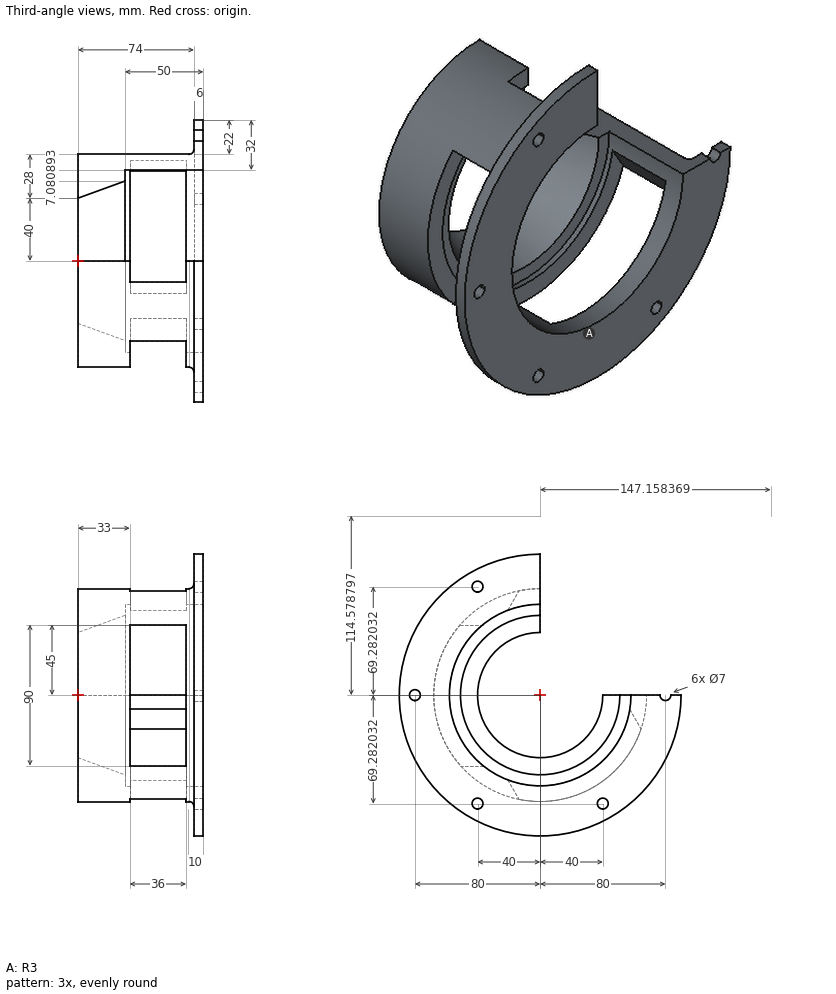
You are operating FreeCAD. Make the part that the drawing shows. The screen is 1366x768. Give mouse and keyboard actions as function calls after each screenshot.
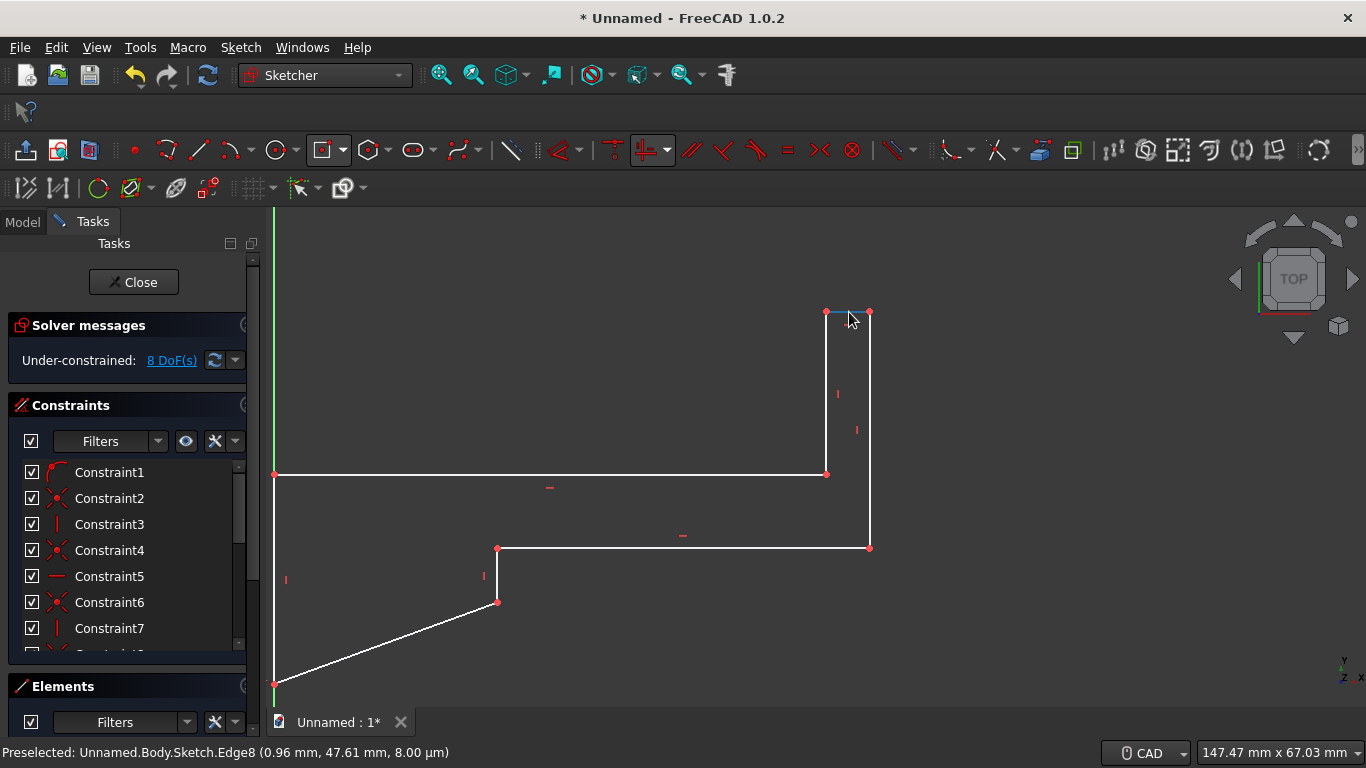
click(848, 312)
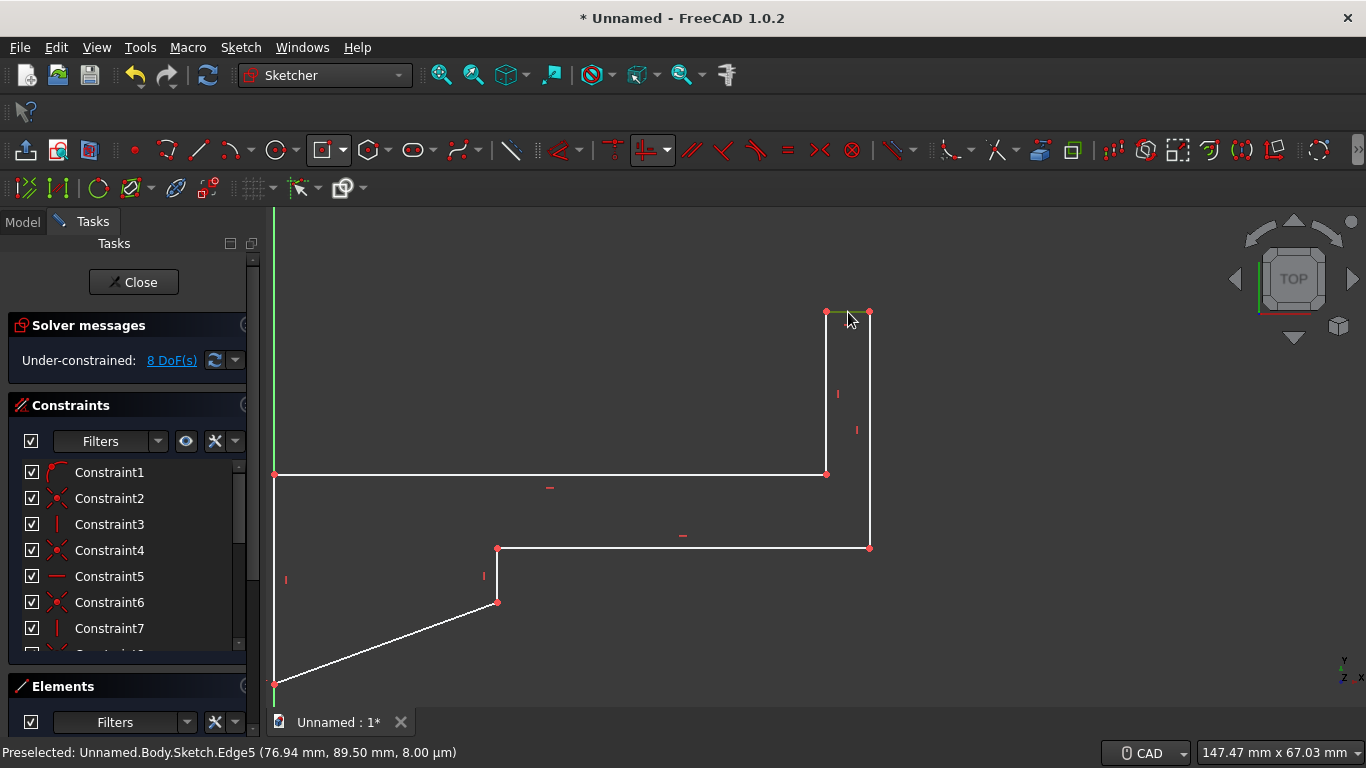
key(l)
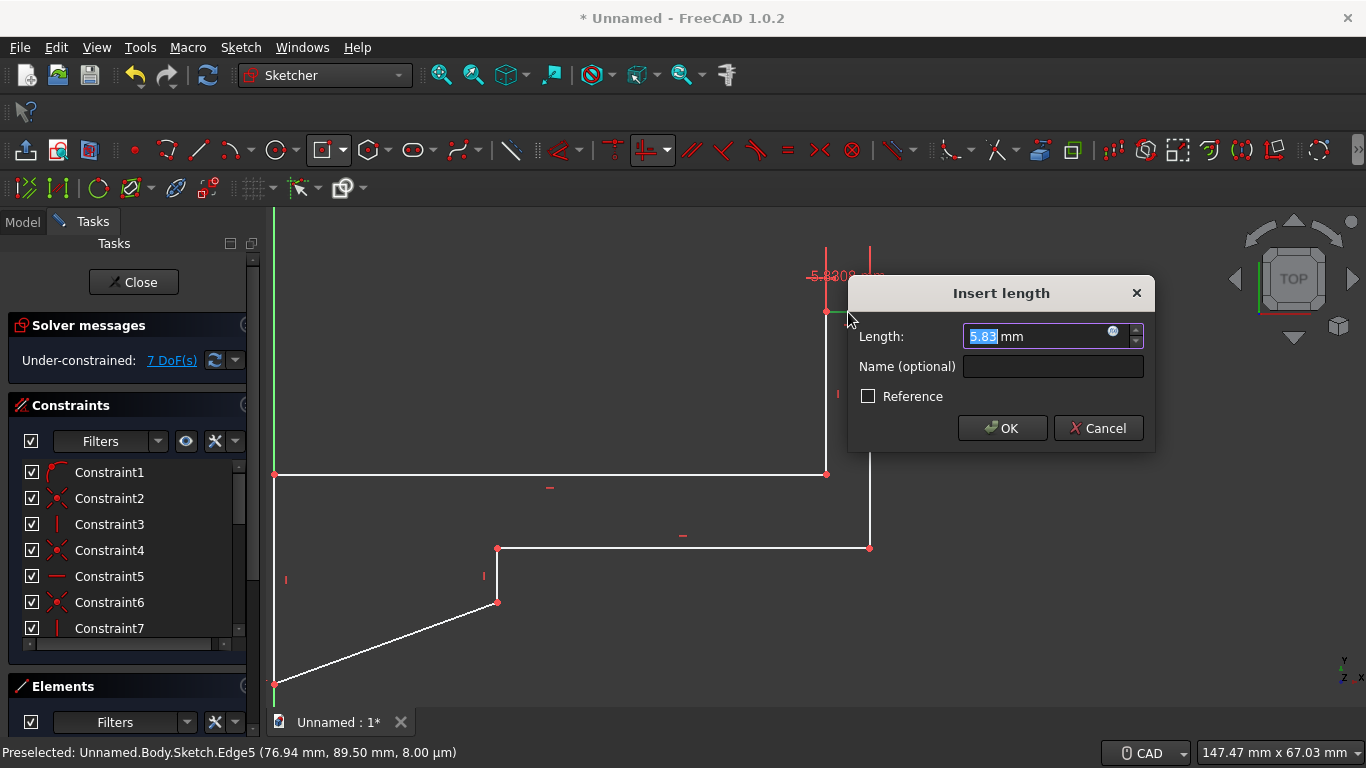
text(6)
key(Return)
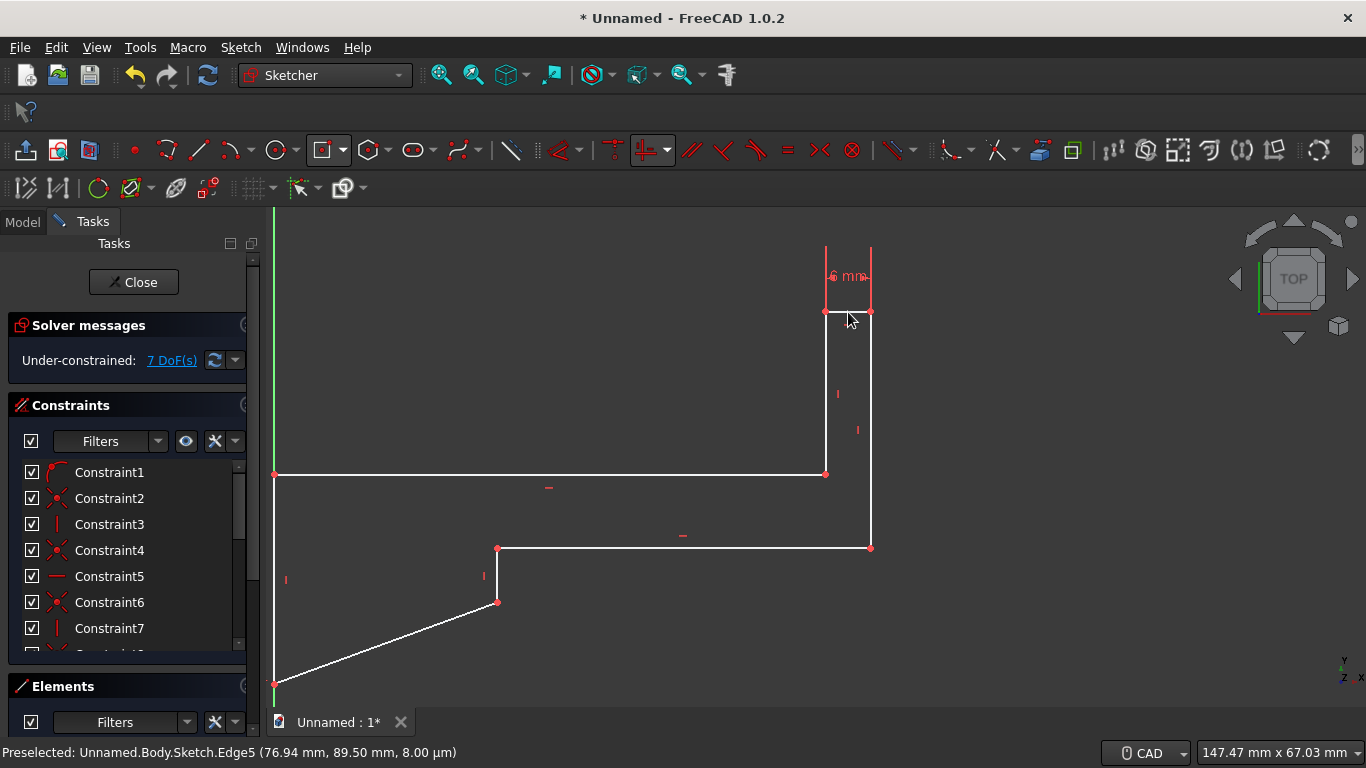
click(609, 548)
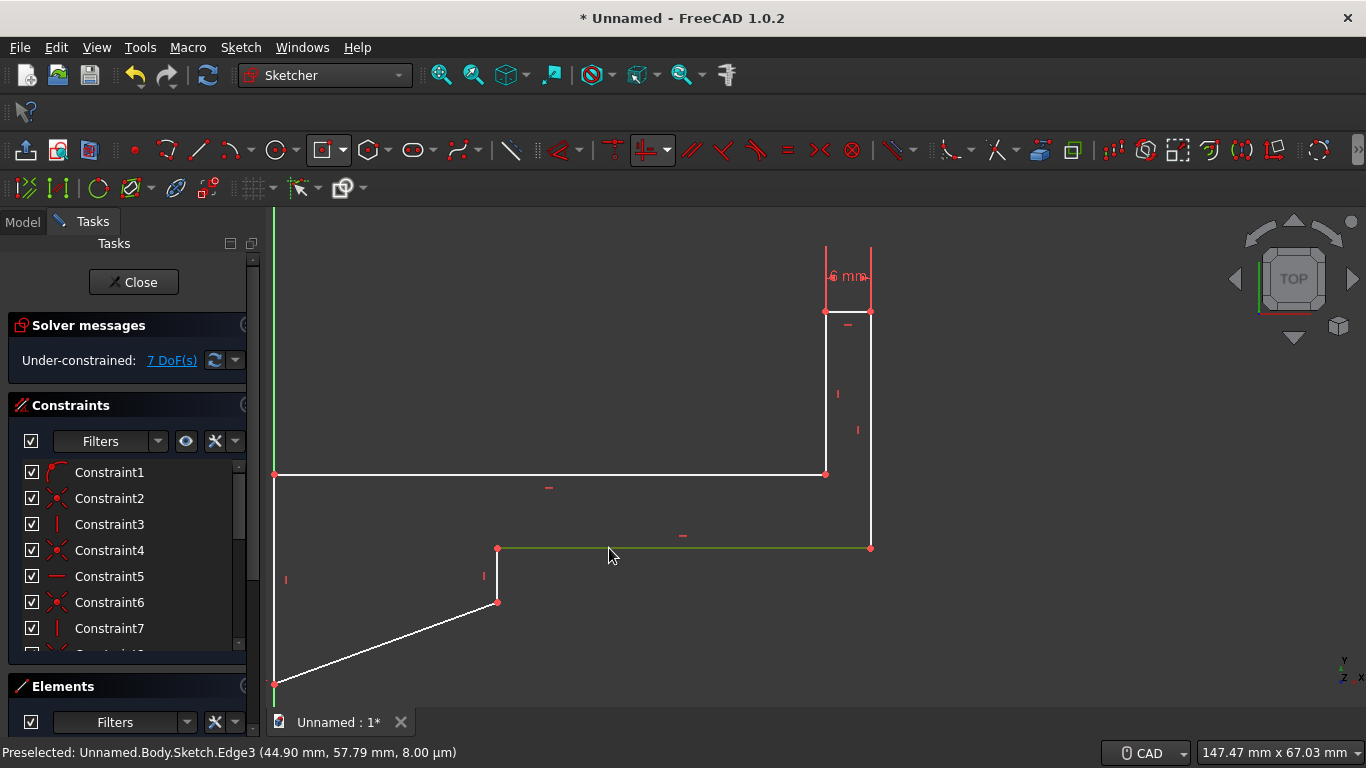
key(l)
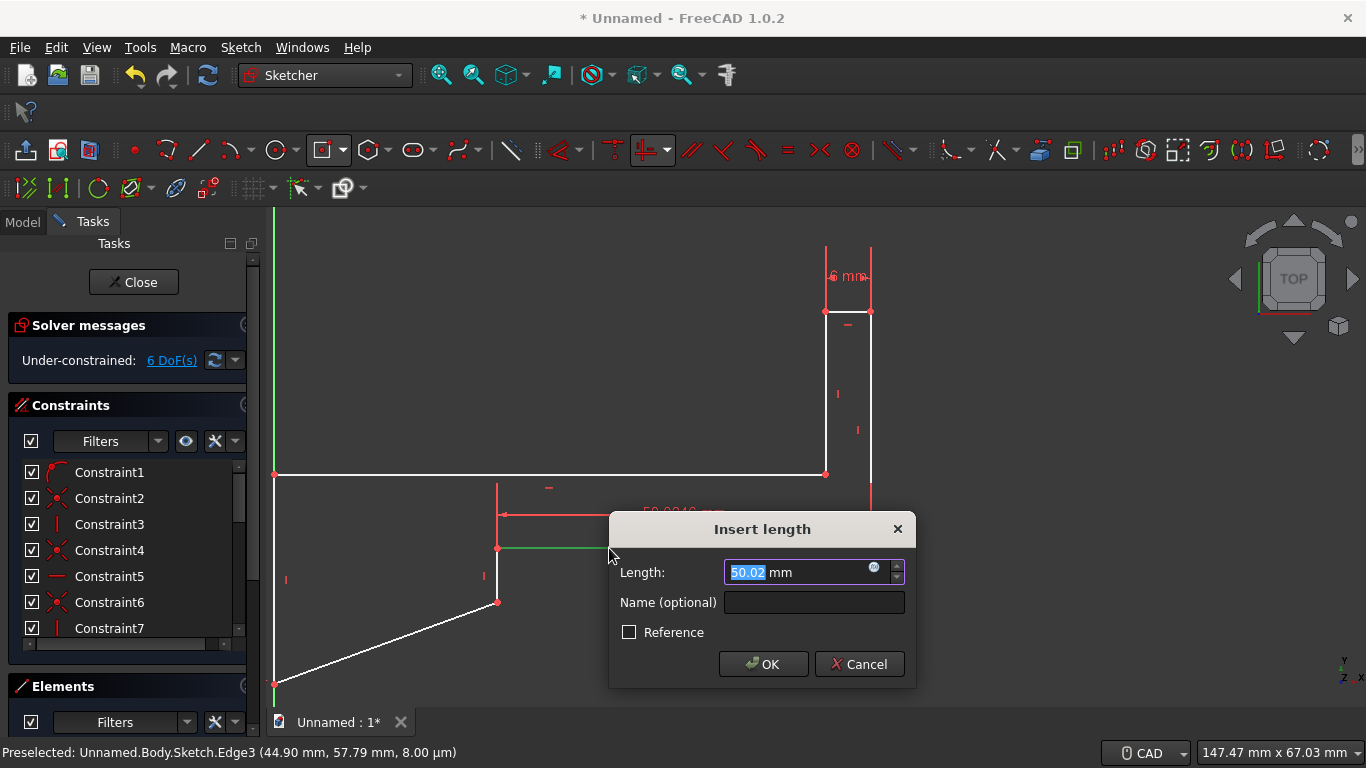
text(50)
key(Return)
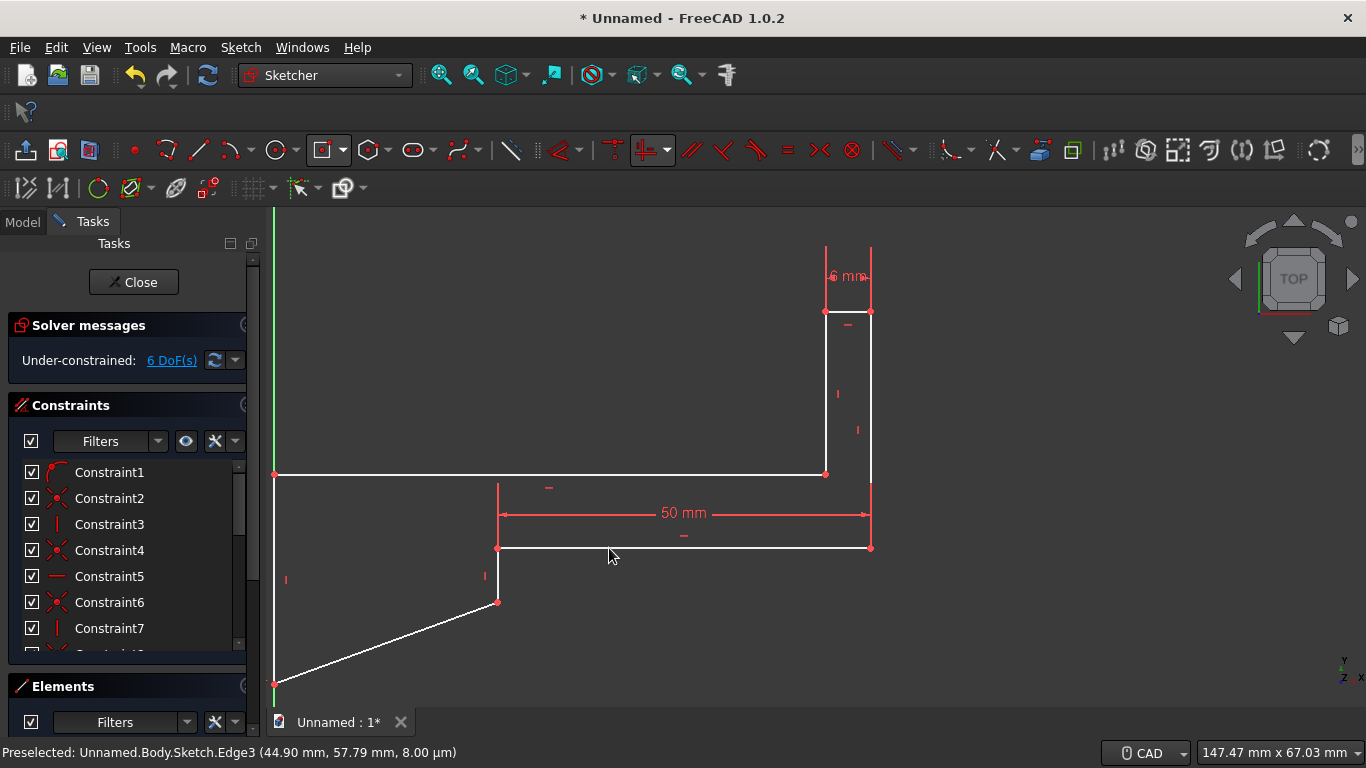
click(871, 477)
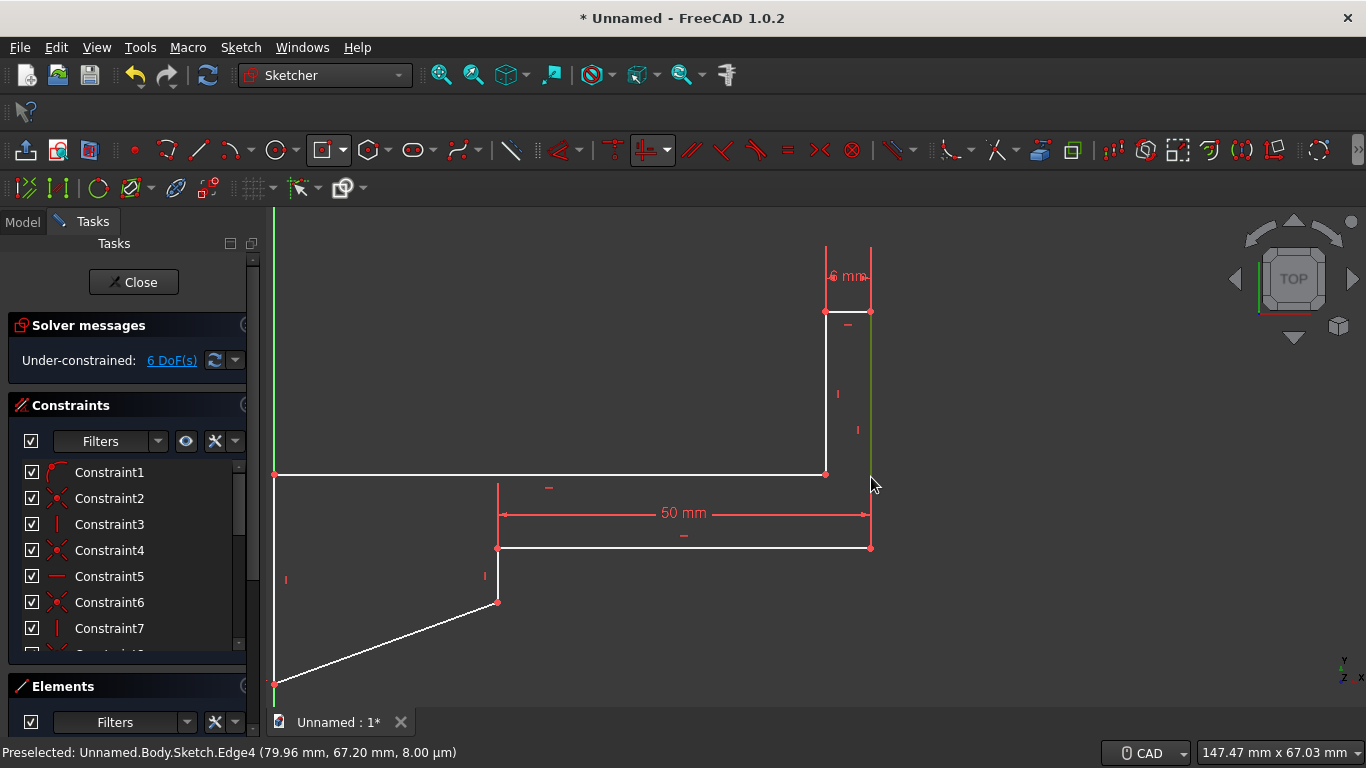
key(i)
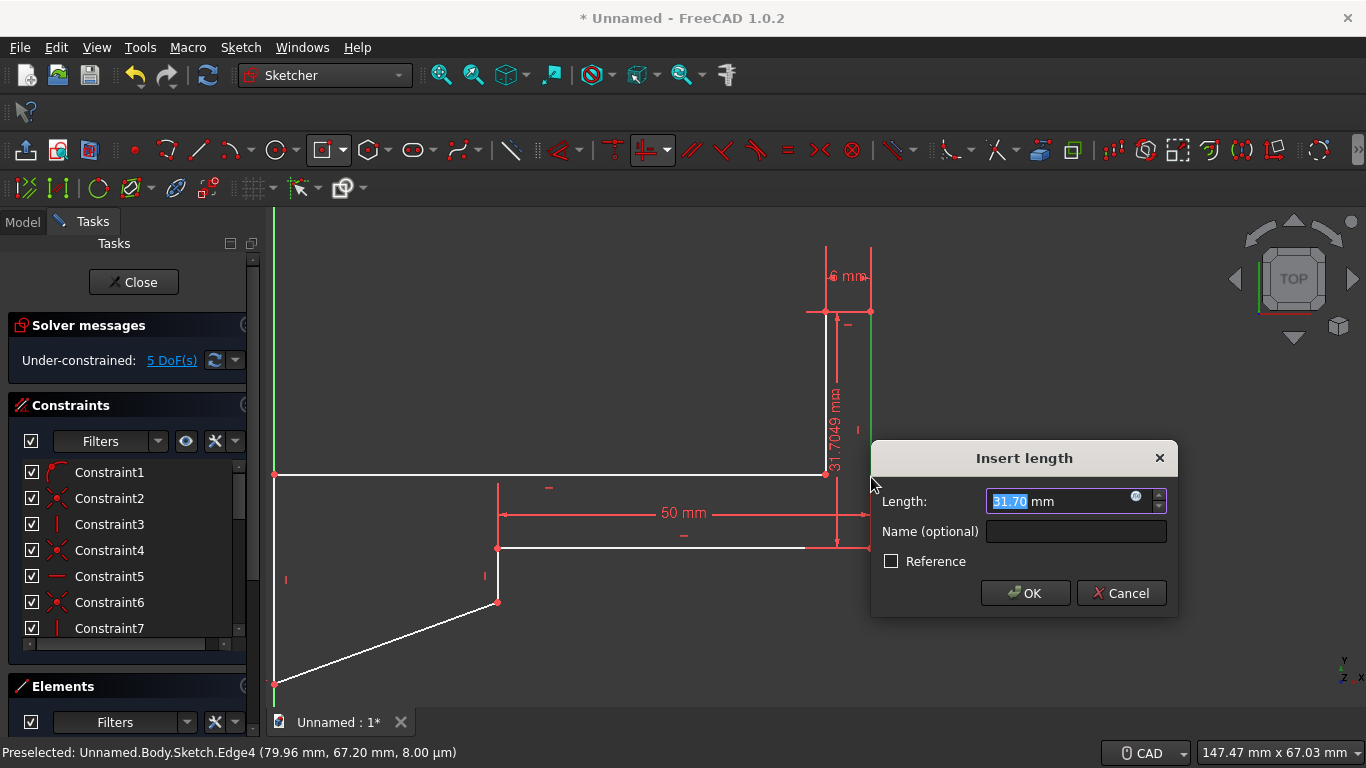
text(32)
key(Return)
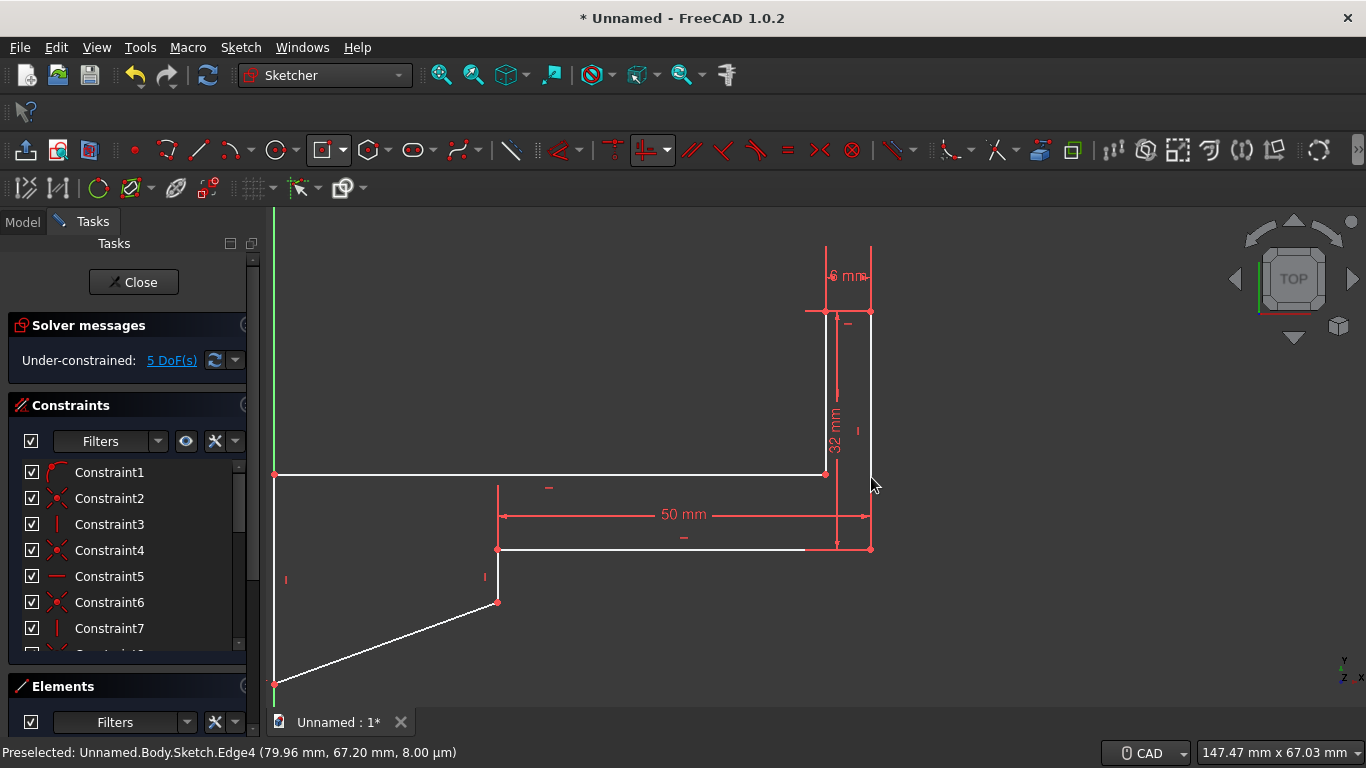
click(826, 360)